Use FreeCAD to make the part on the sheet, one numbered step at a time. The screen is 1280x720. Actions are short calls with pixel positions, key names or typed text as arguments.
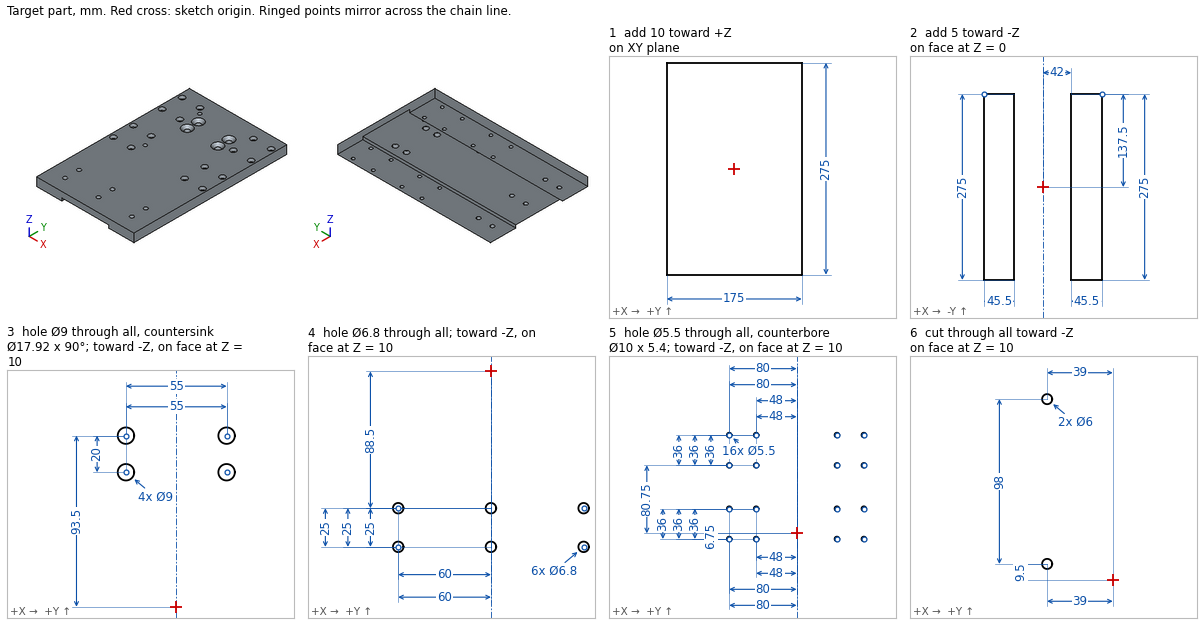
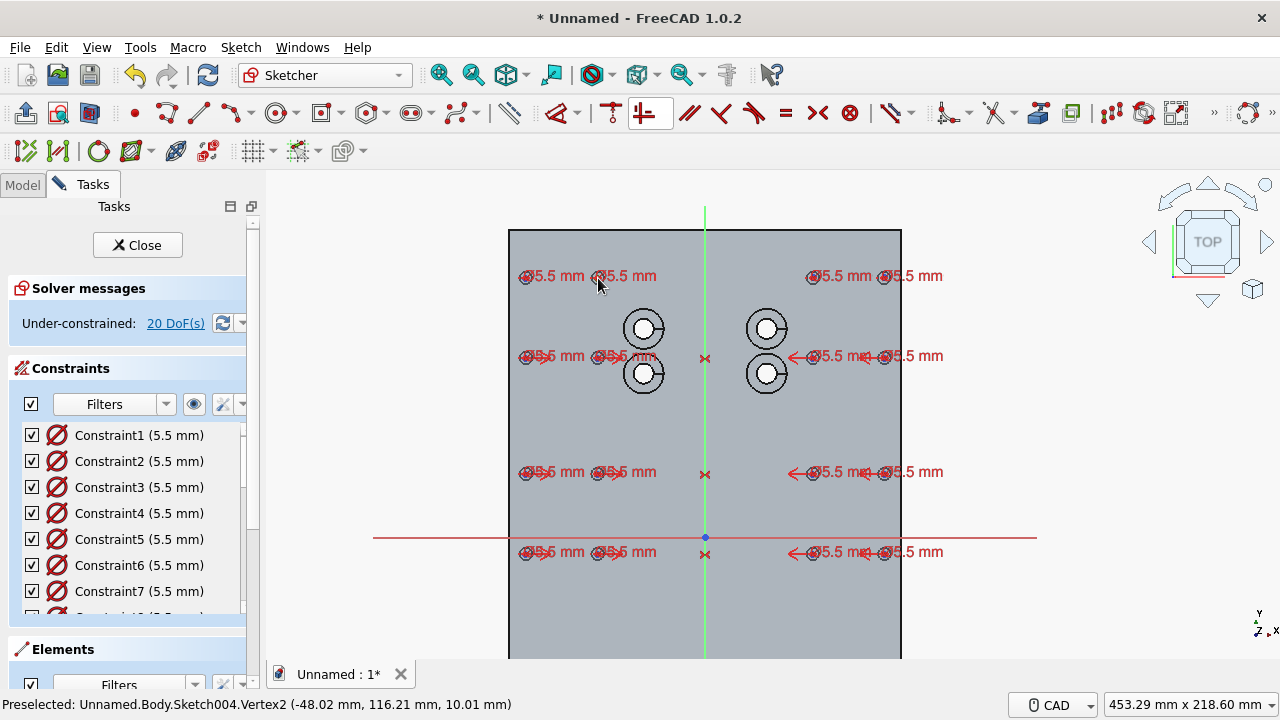
click(813, 278)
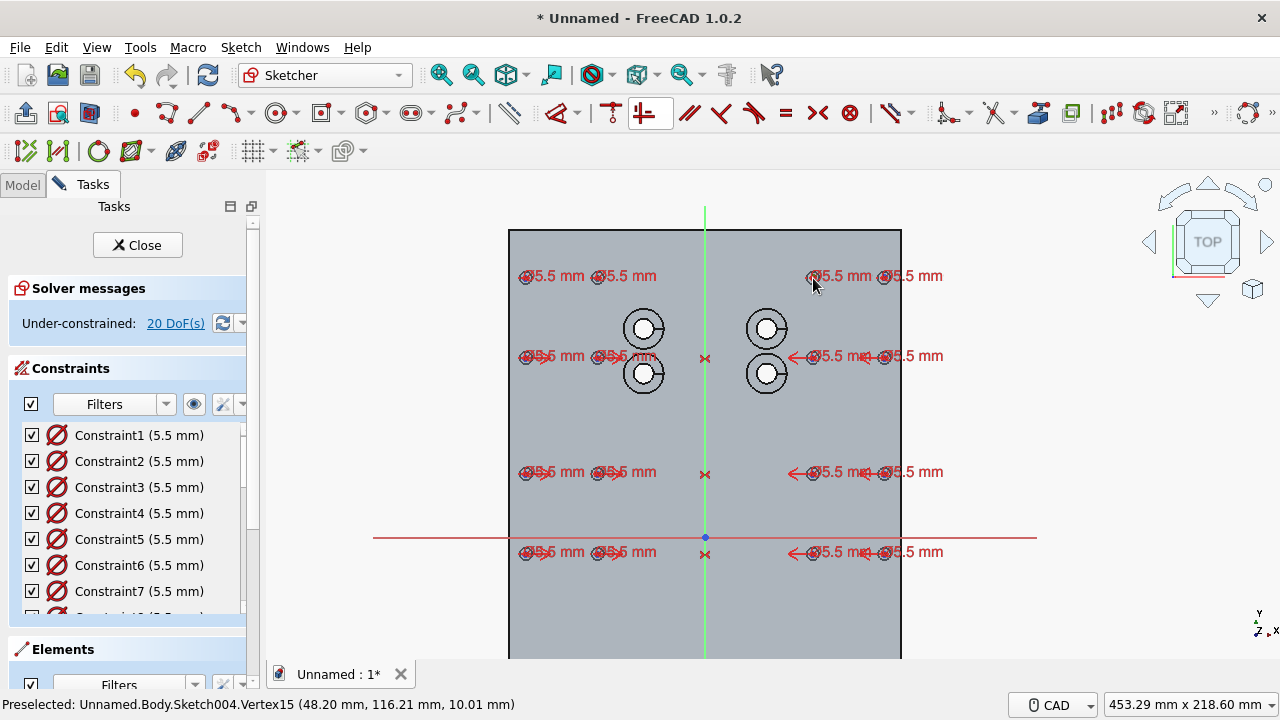
click(705, 600)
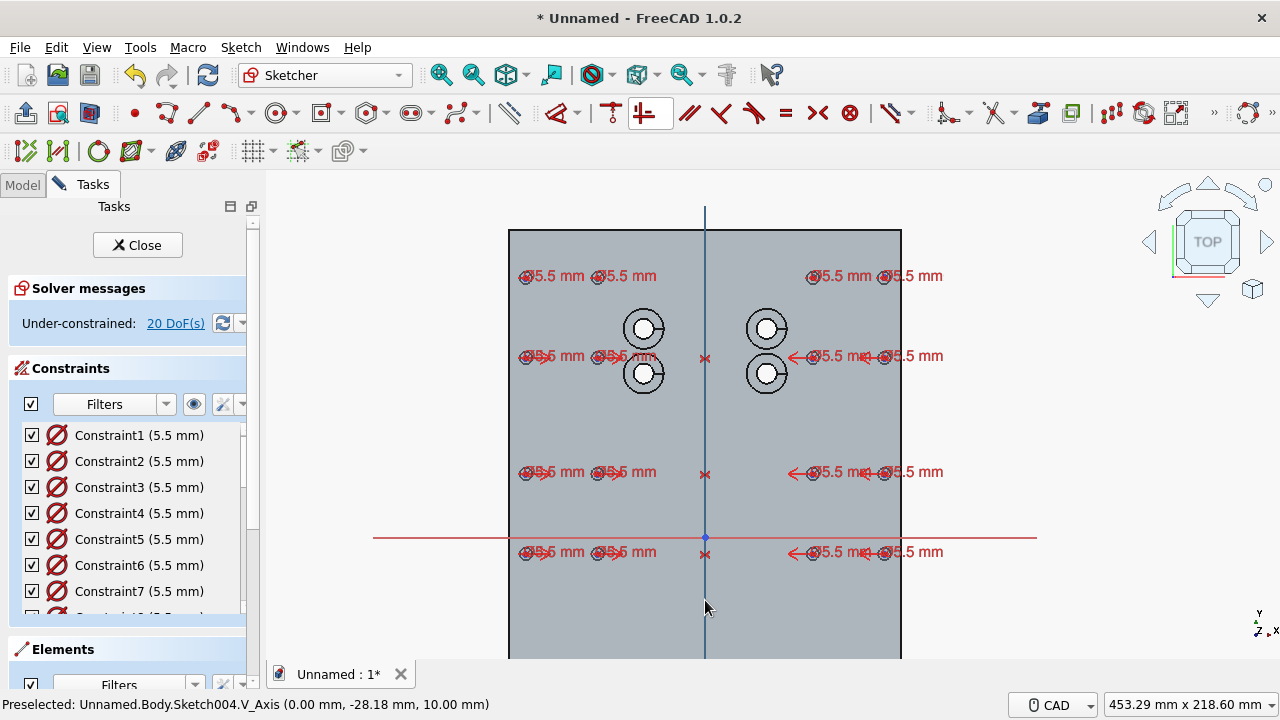
click(818, 114)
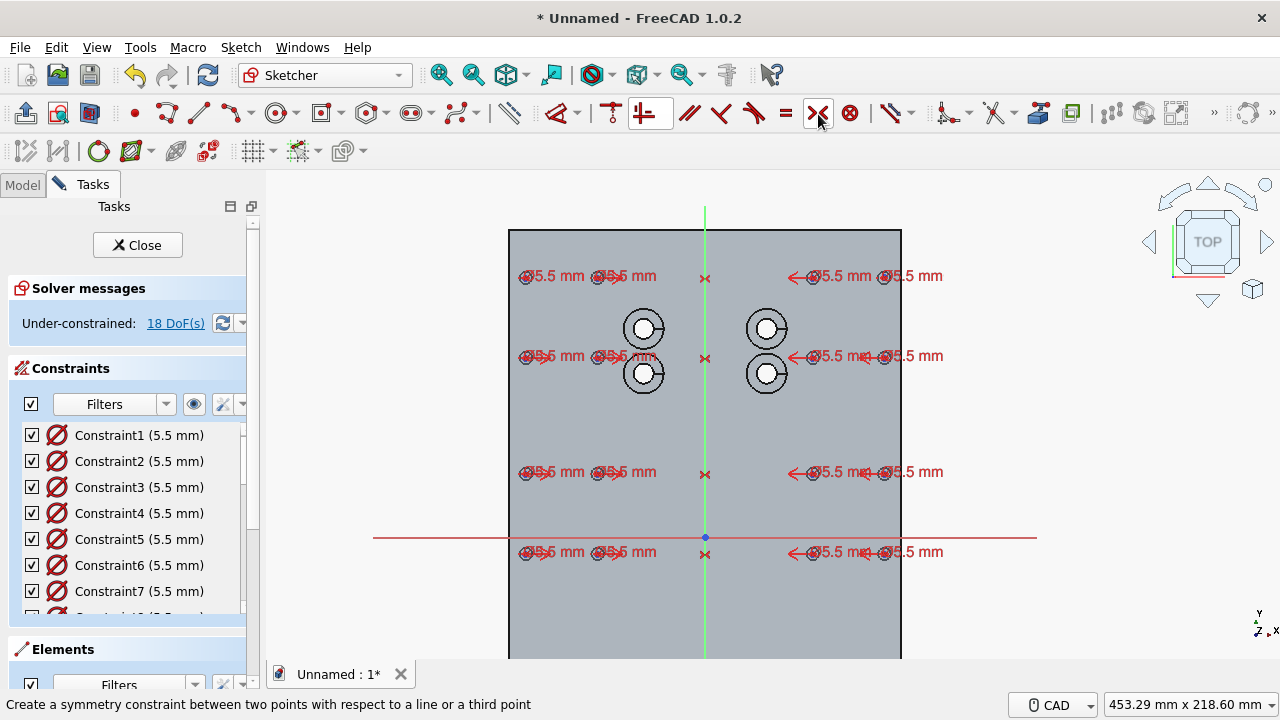
click(526, 278)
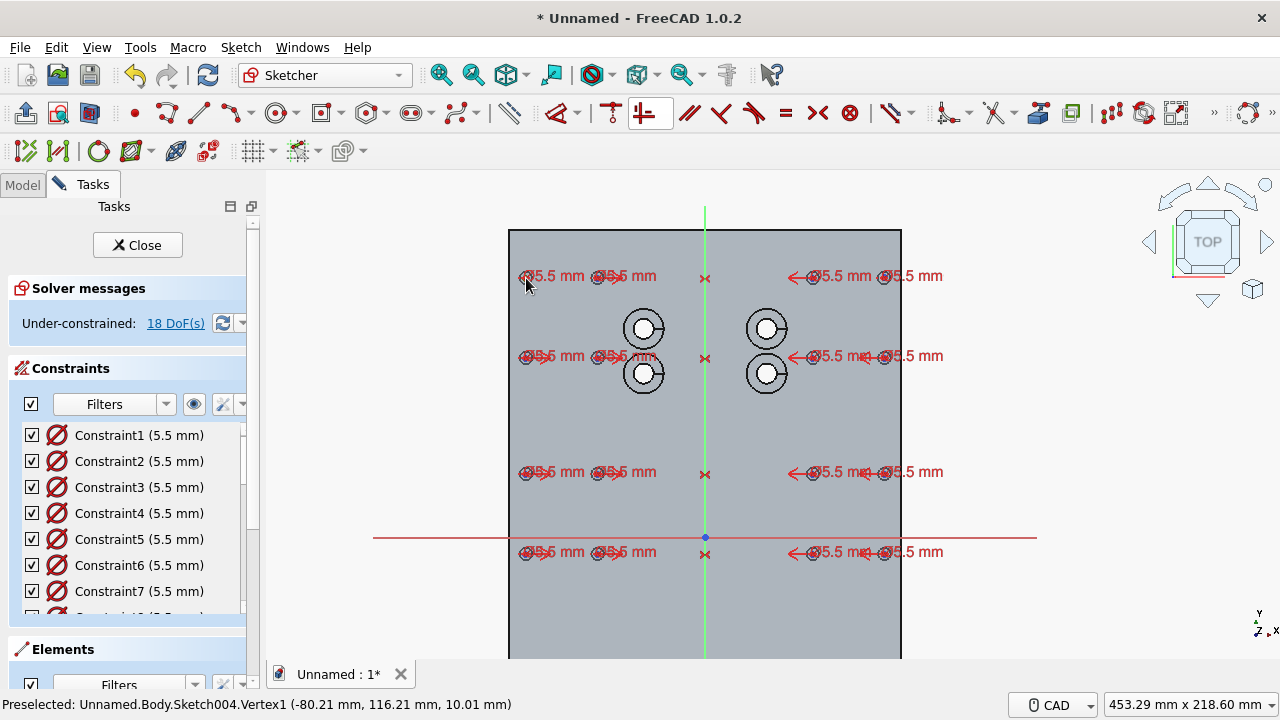
click(884, 278)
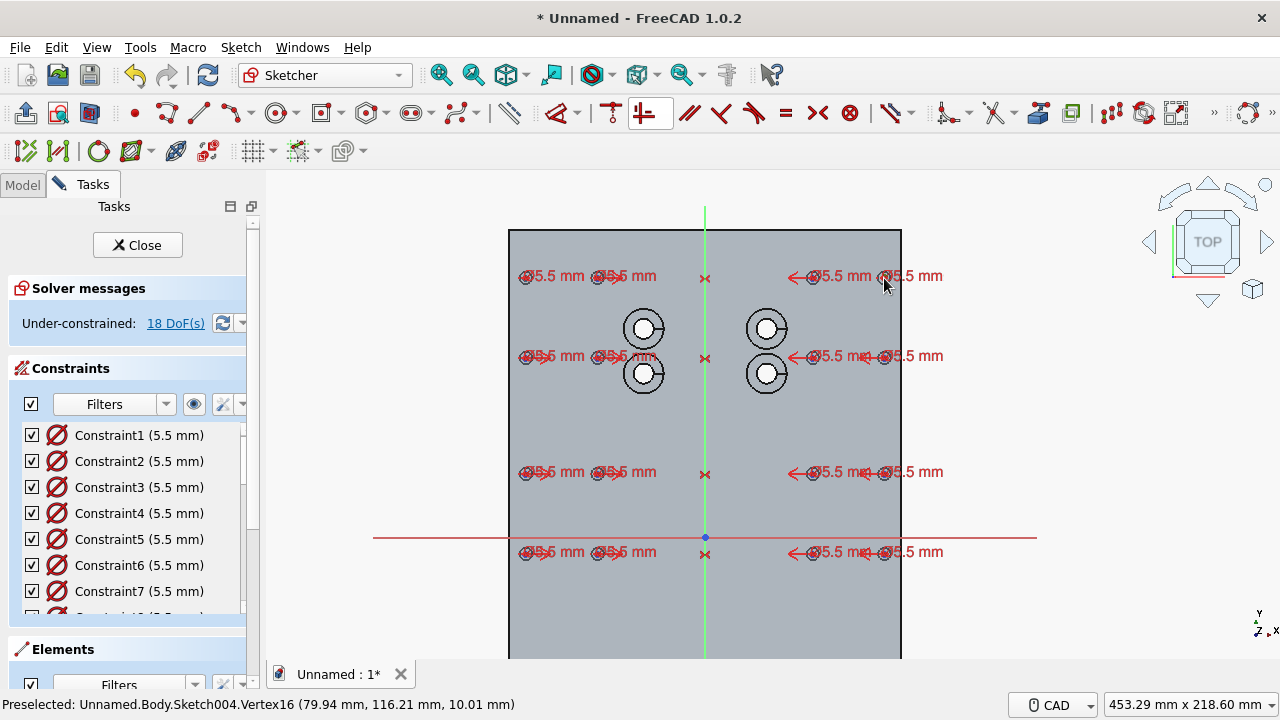
click(705, 600)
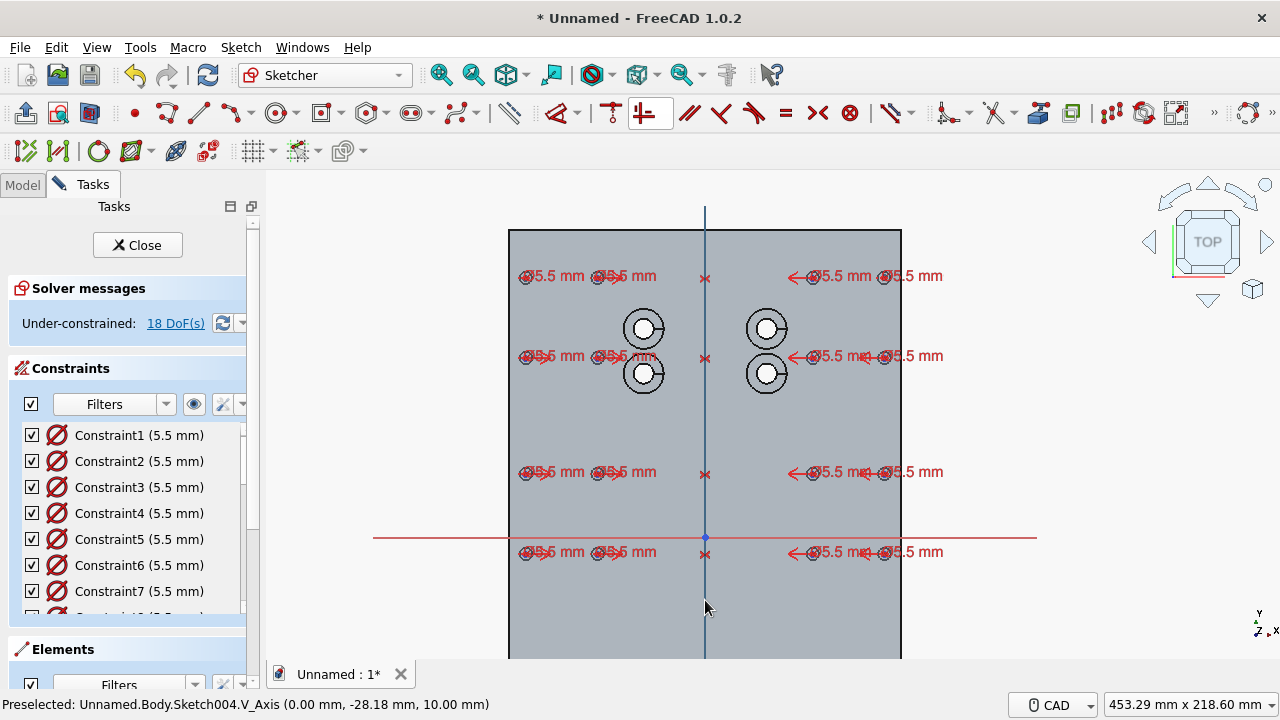
key(s)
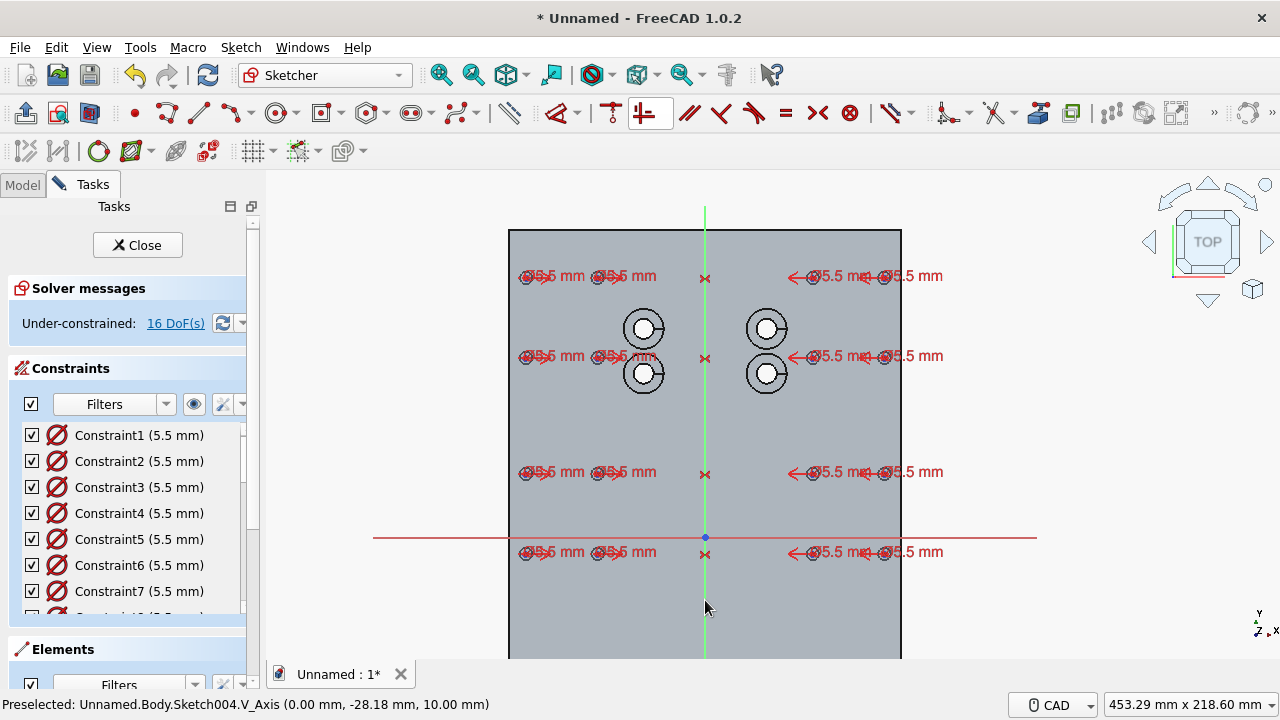
key(d)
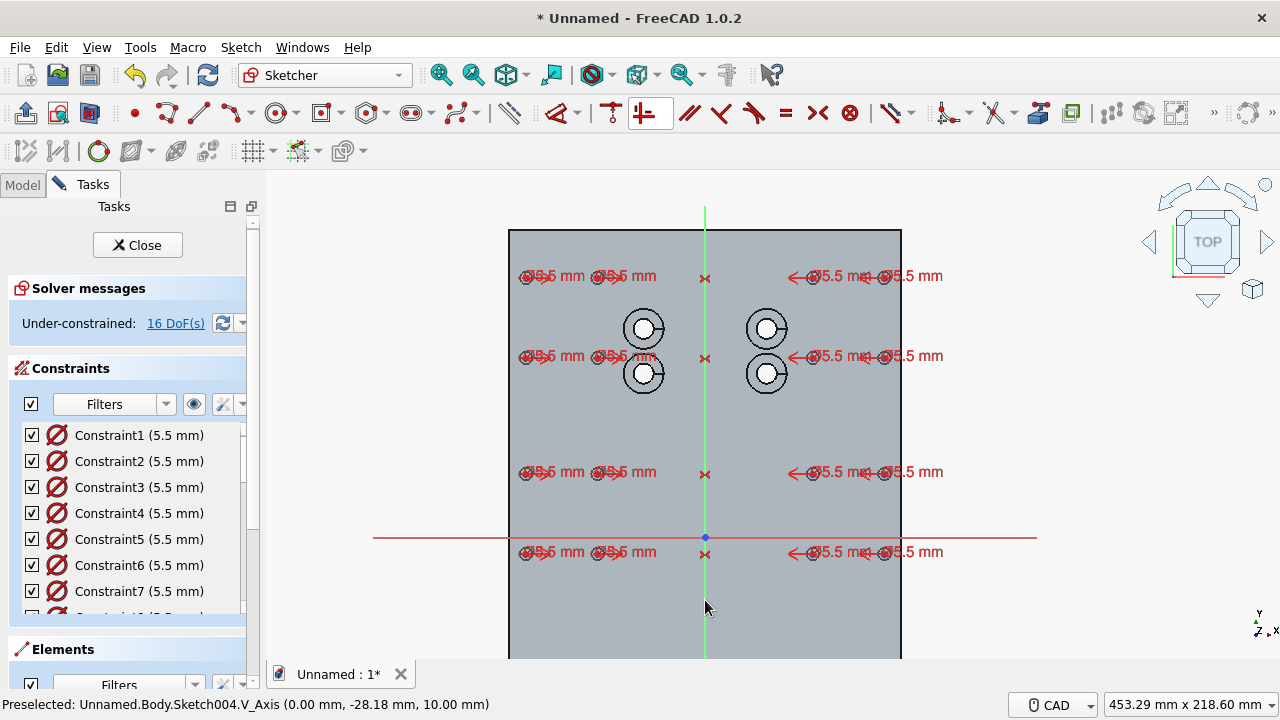
click(526, 278)
click(616, 244)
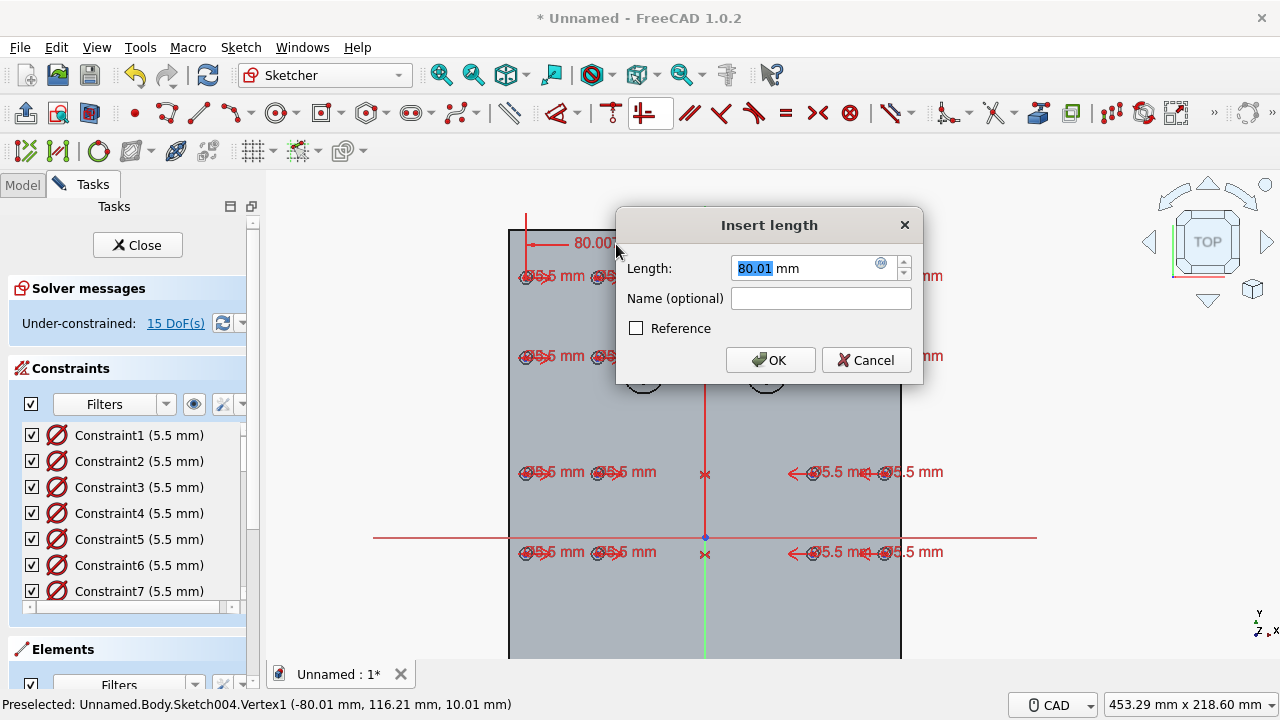
text(80)
key(Return)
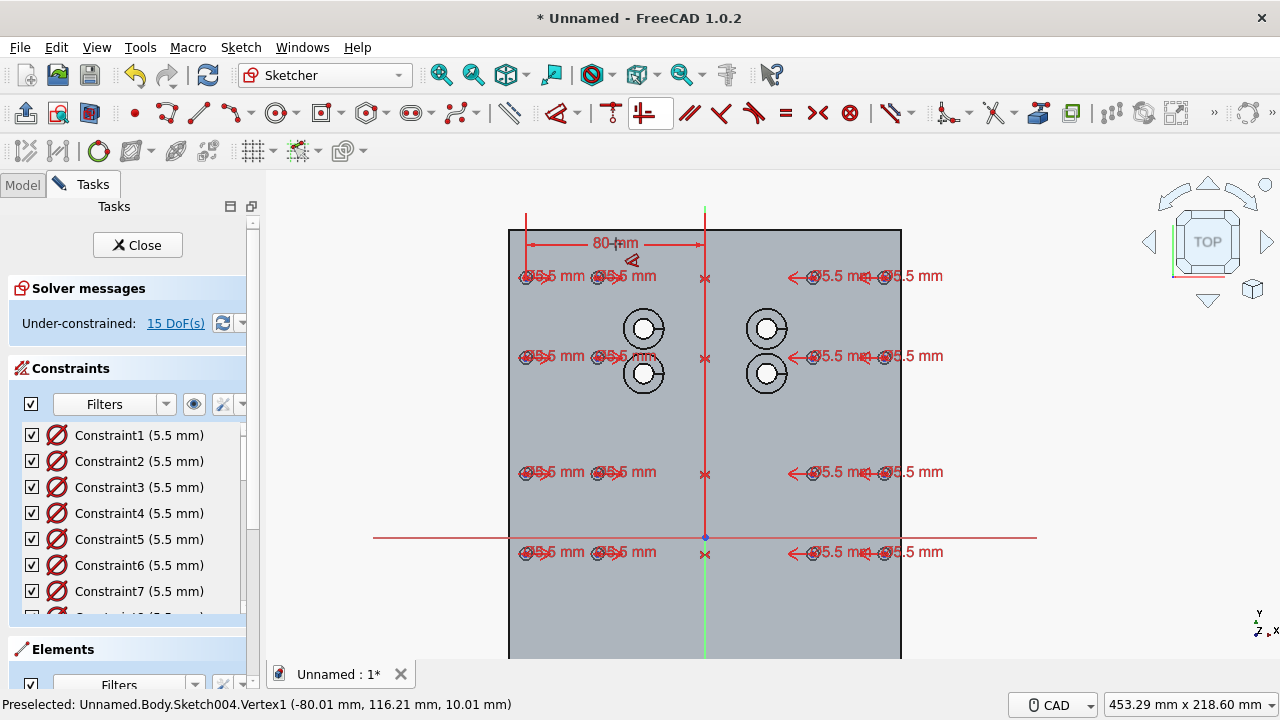
click(598, 278)
click(689, 244)